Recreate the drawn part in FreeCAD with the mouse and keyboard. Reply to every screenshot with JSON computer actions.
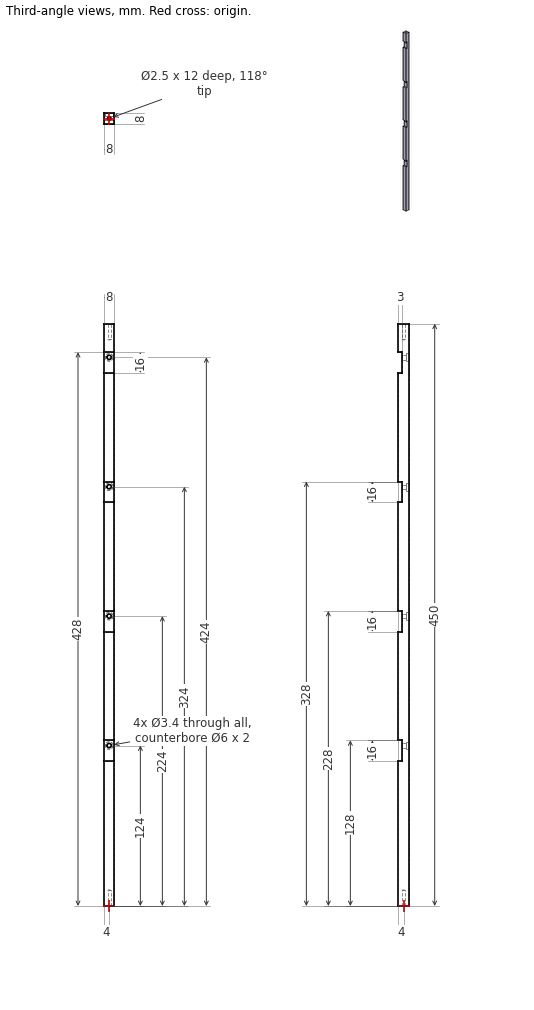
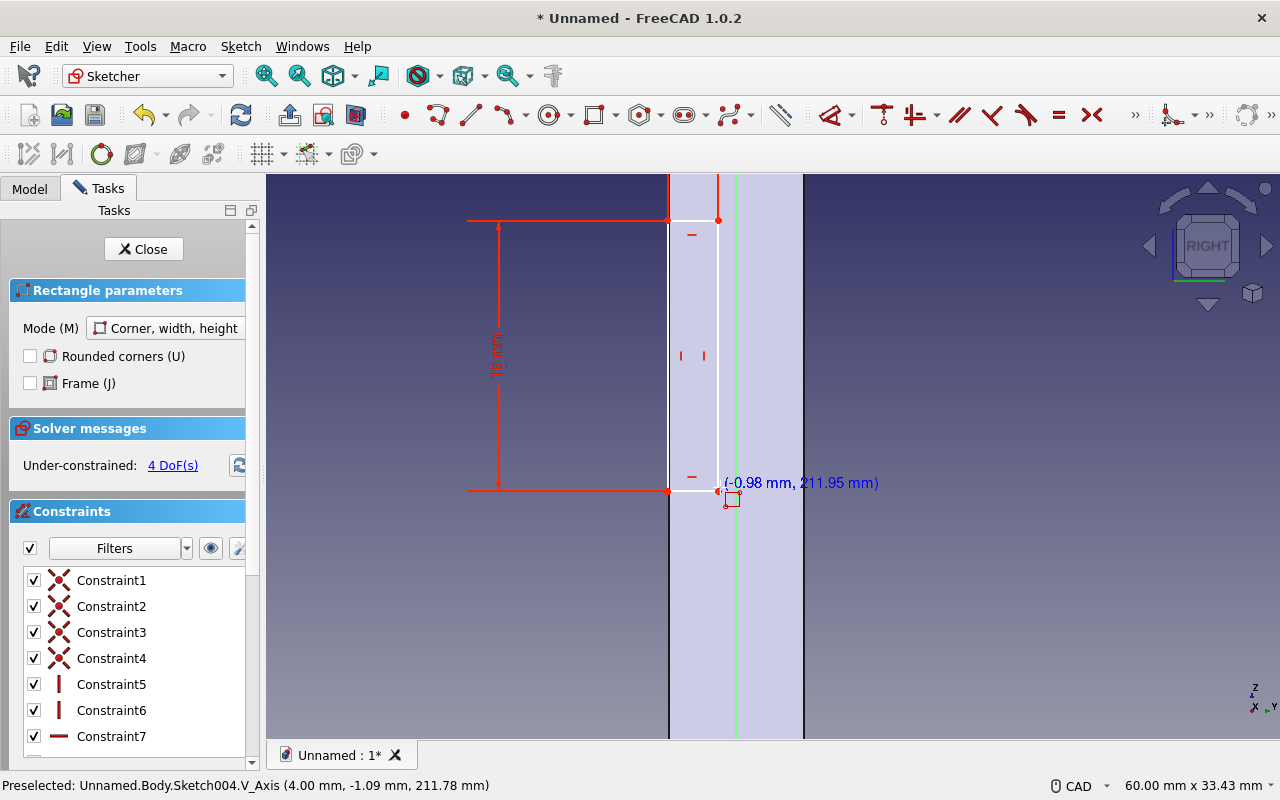
{"action": "scroll", "coordinate": [705, 402], "scroll_direction": "down", "scroll_amount": 14}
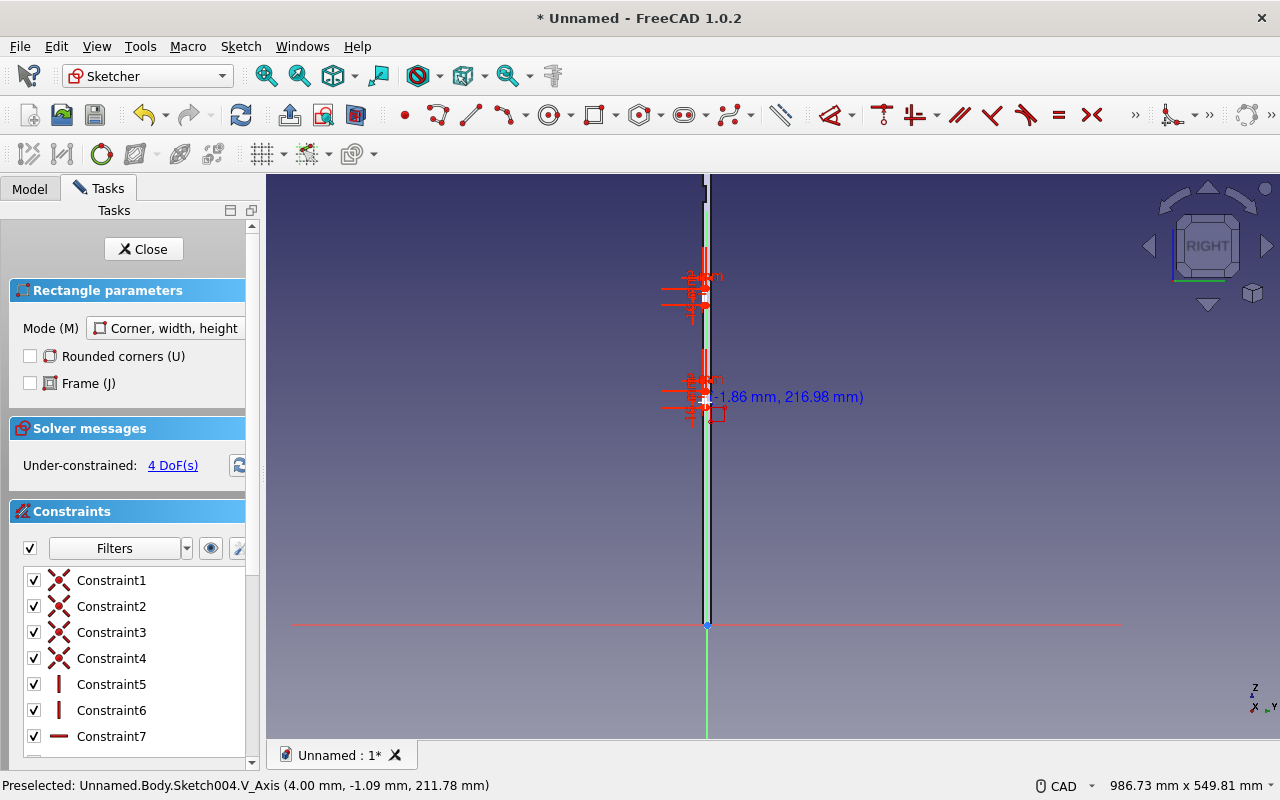
{"action": "scroll", "coordinate": [703, 494], "scroll_direction": "up", "scroll_amount": 9}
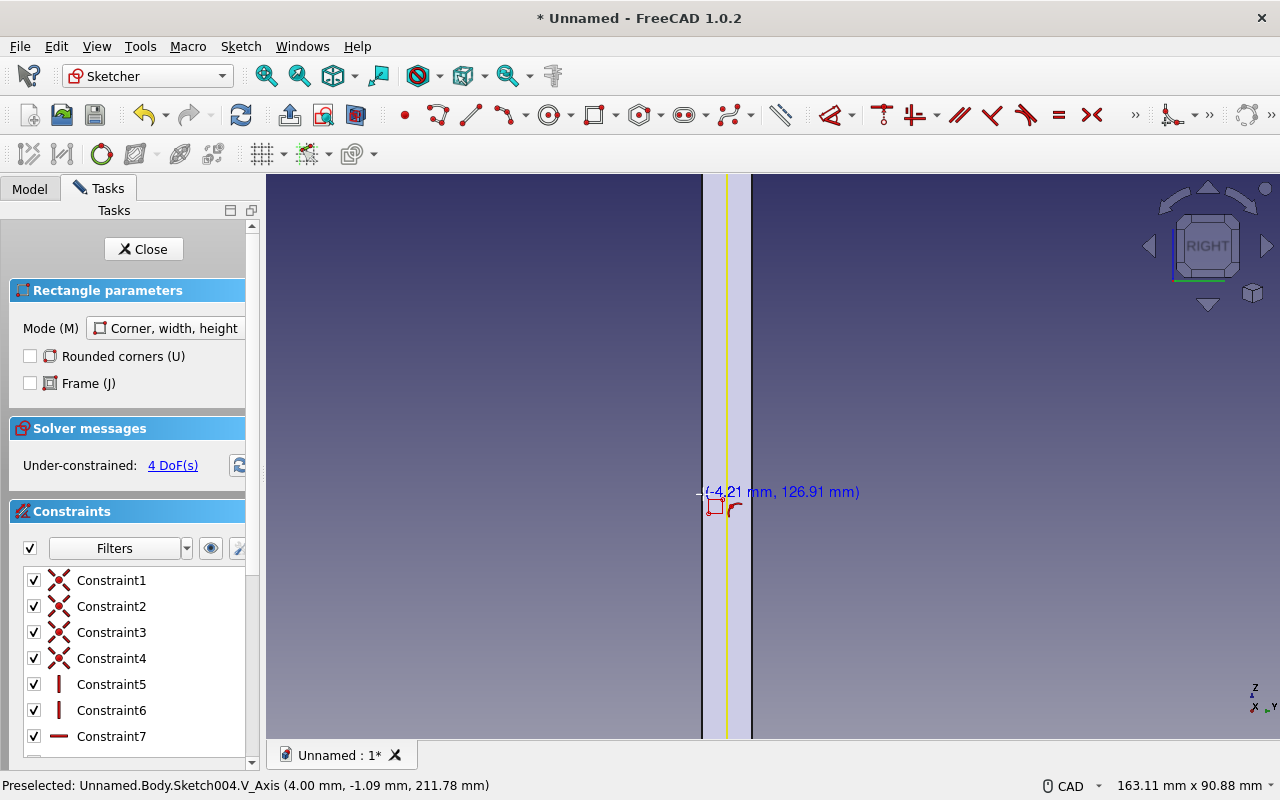
{"action": "left_click", "coordinate": [702, 490]}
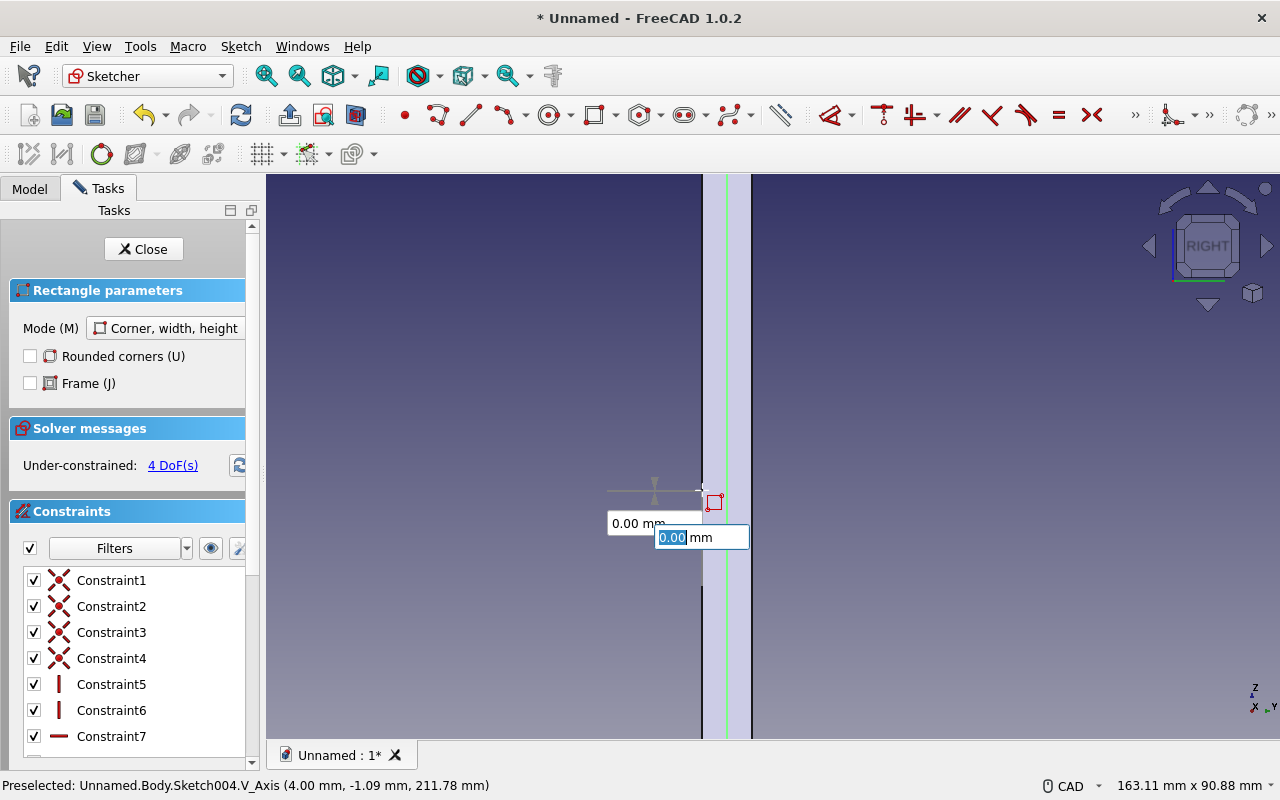
{"action": "scroll", "coordinate": [721, 590], "scroll_direction": "up", "scroll_amount": 5}
{"action": "mouse_move", "coordinate": [720, 588]}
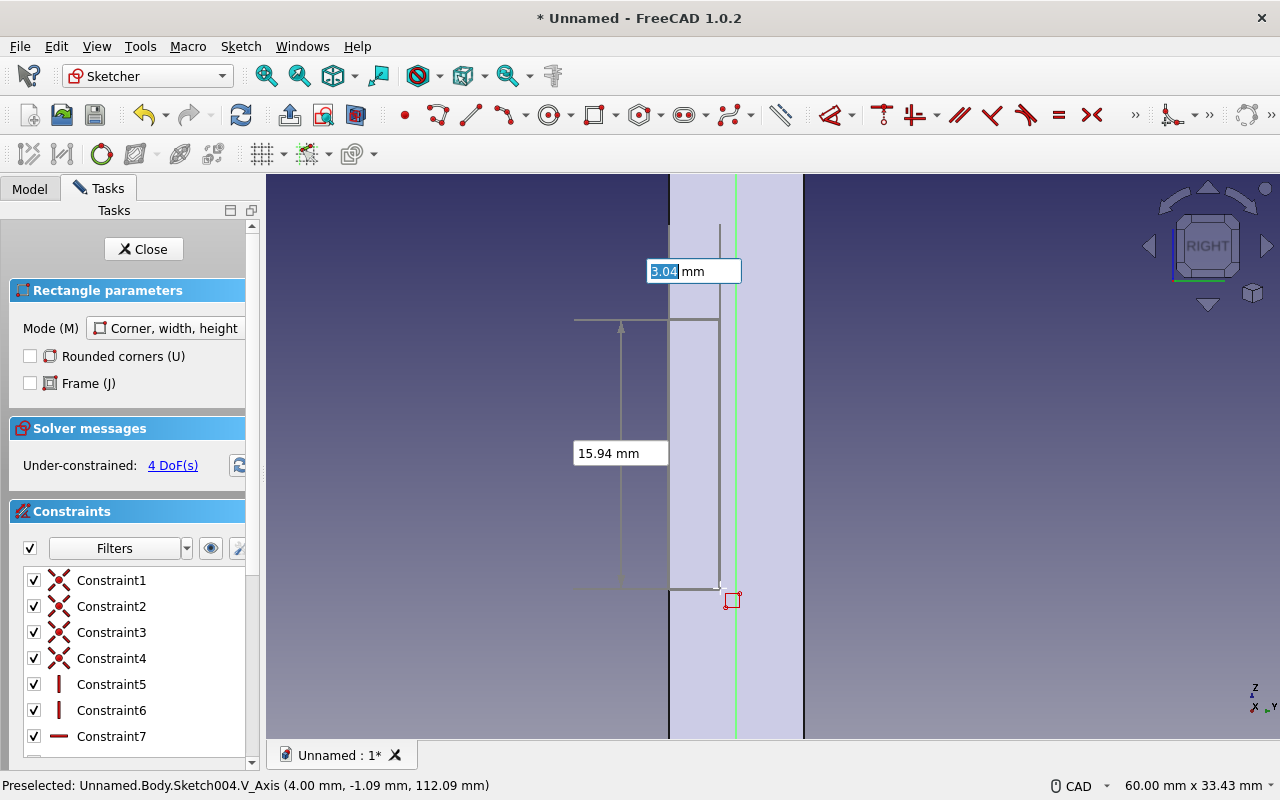
{"action": "type", "text": "3"}
{"action": "key", "text": "Tab"}
{"action": "type", "text": "16"}
{"action": "key", "text": "Return"}
{"action": "key", "text": "Escape"}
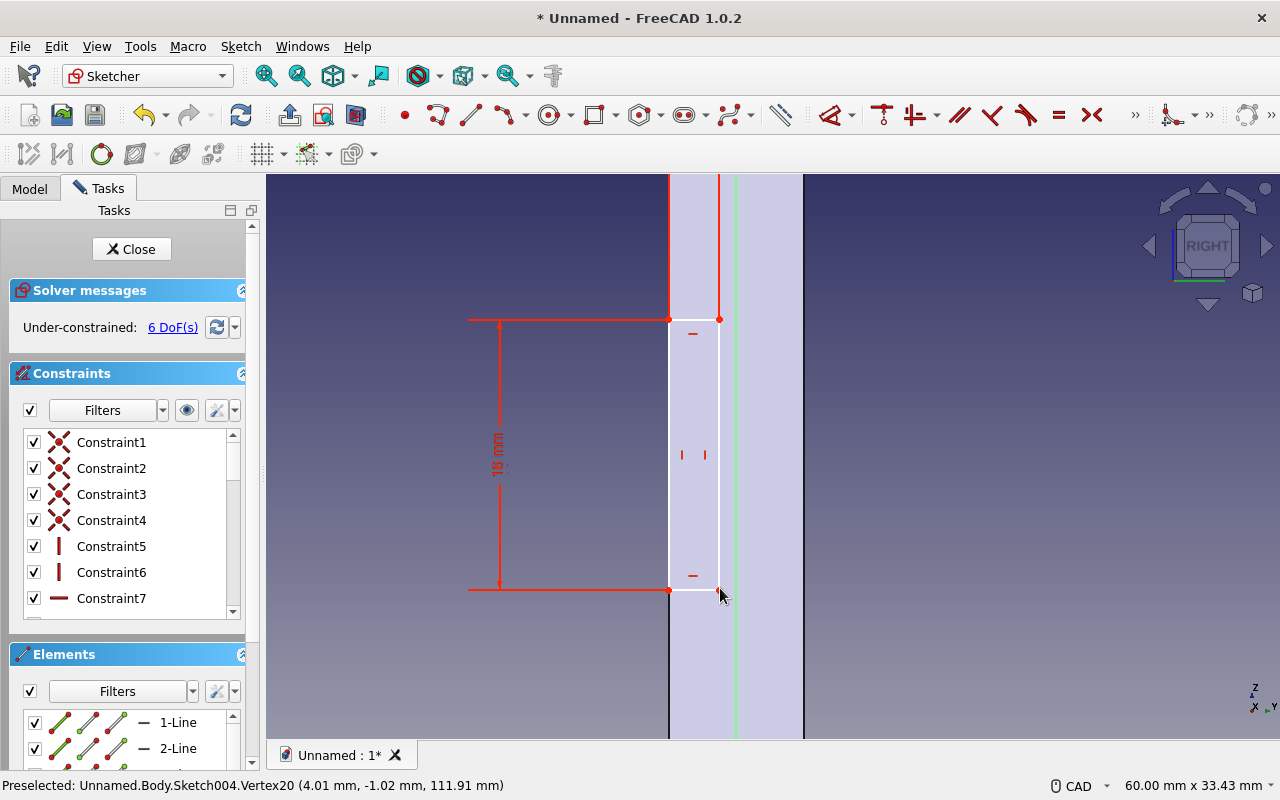
{"action": "key", "text": "d"}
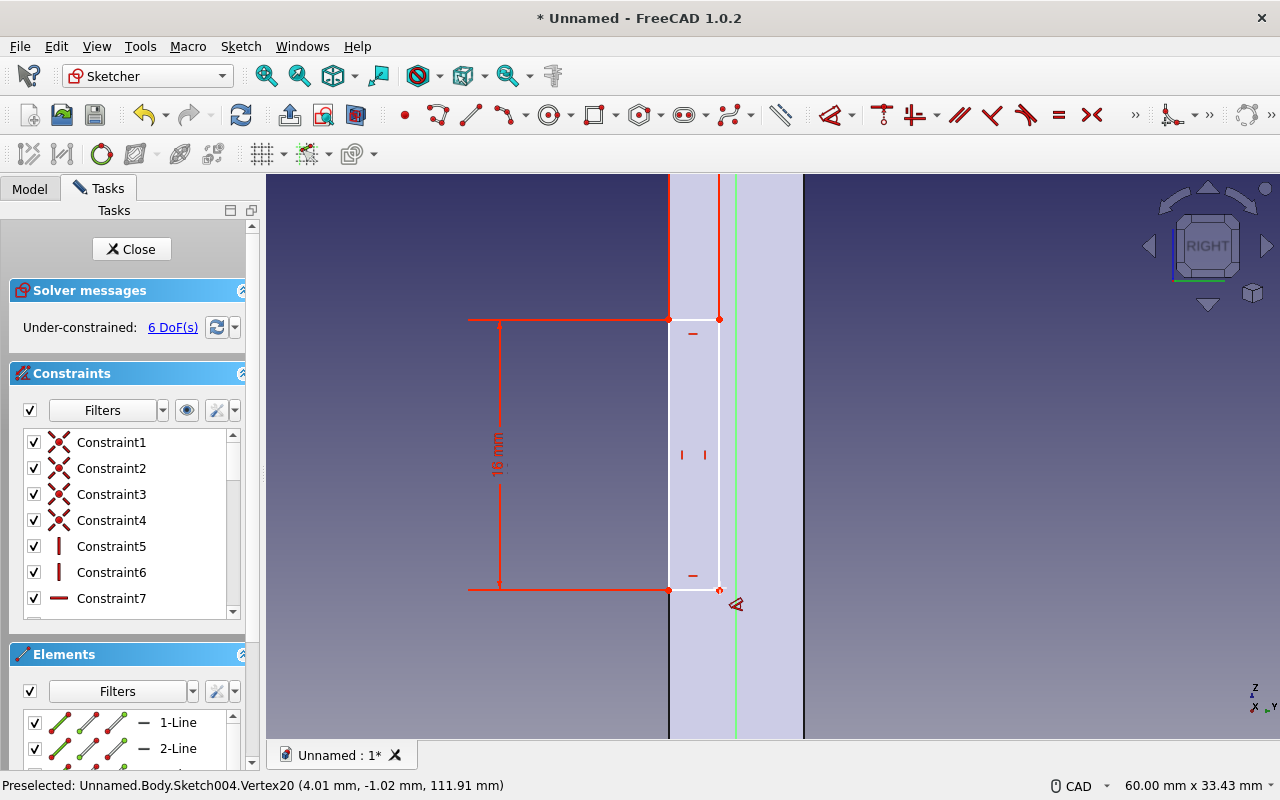
{"action": "scroll", "coordinate": [705, 505], "scroll_direction": "down", "scroll_amount": 14}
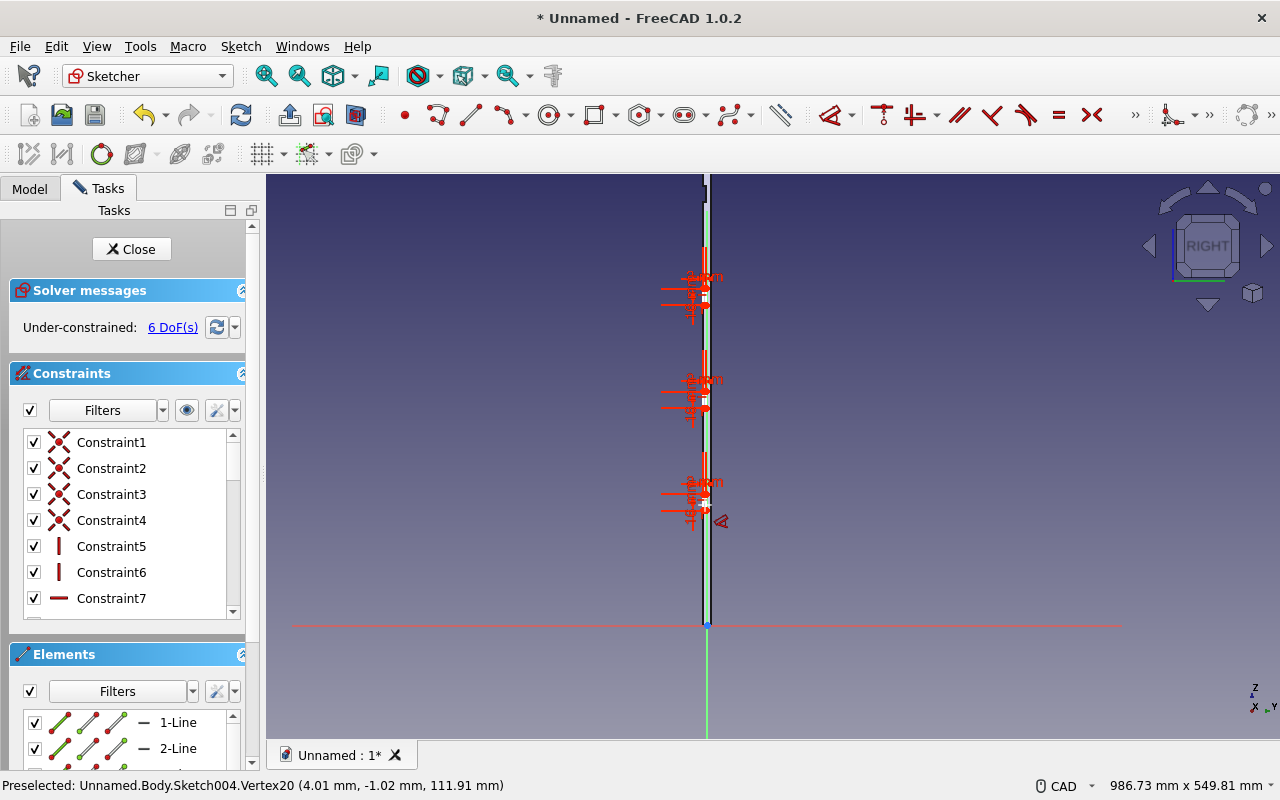
{"action": "scroll", "coordinate": [703, 289], "scroll_direction": "up", "scroll_amount": 12}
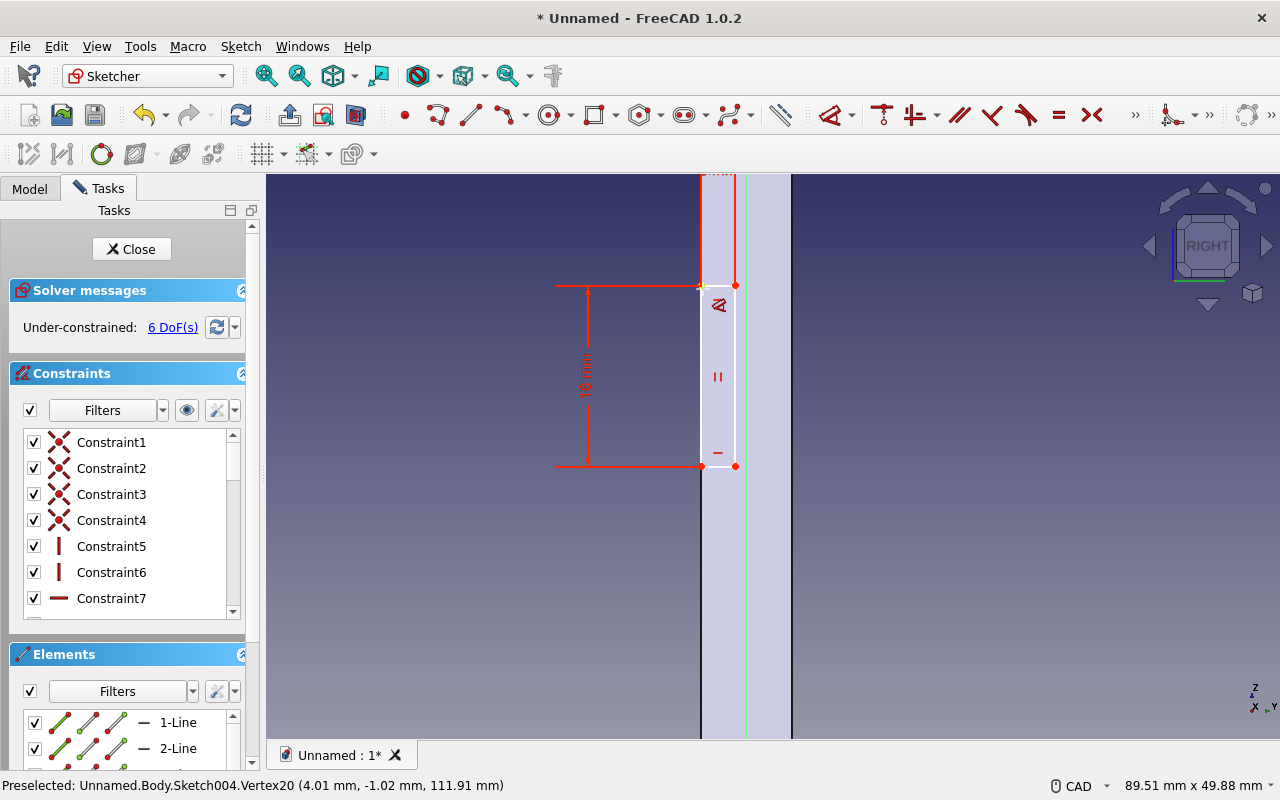
{"action": "left_click", "coordinate": [701, 286]}
{"action": "left_click", "coordinate": [724, 252]}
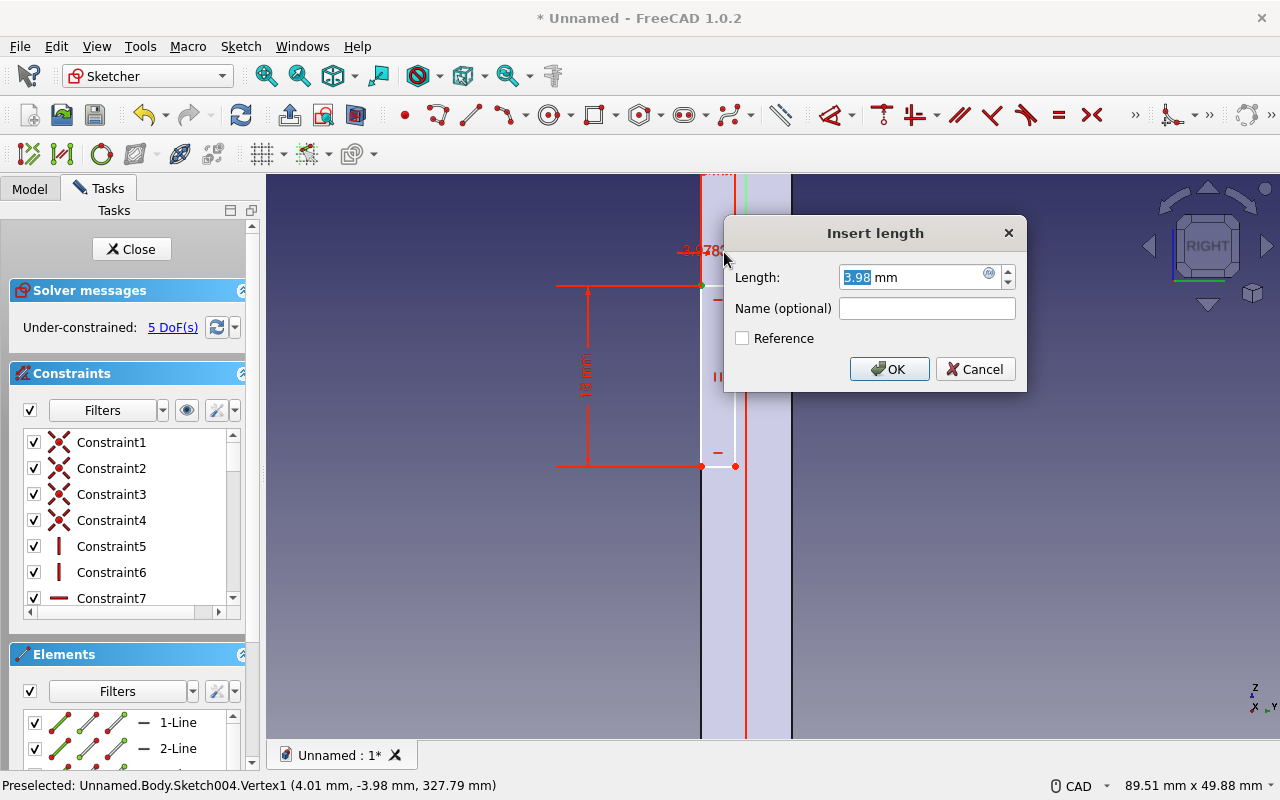
{"action": "type", "text": "4"}
{"action": "key", "text": "Return"}